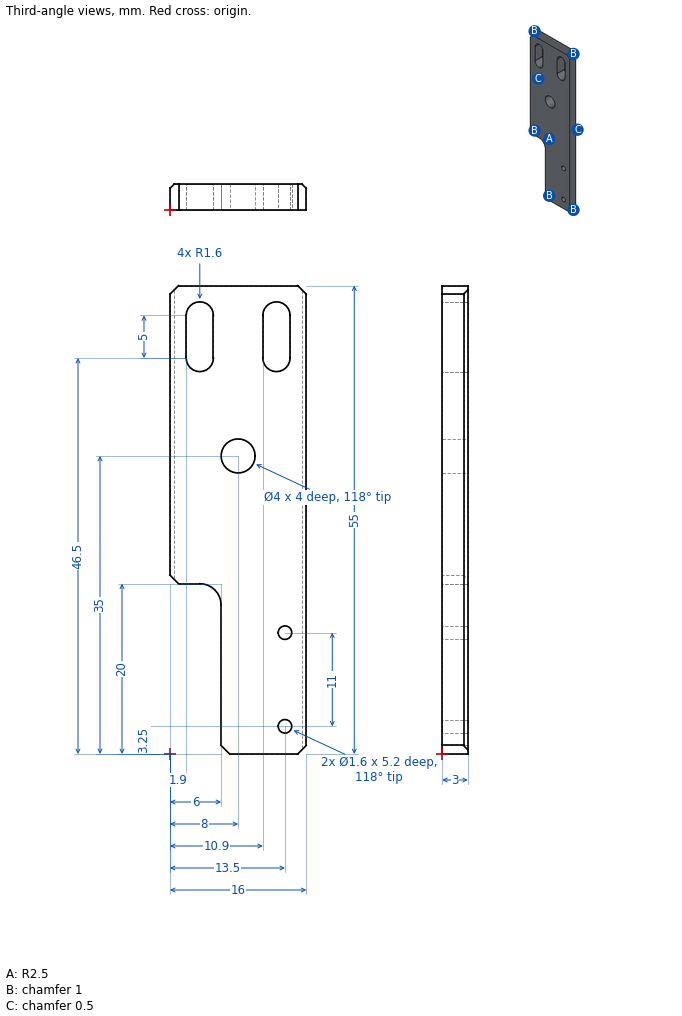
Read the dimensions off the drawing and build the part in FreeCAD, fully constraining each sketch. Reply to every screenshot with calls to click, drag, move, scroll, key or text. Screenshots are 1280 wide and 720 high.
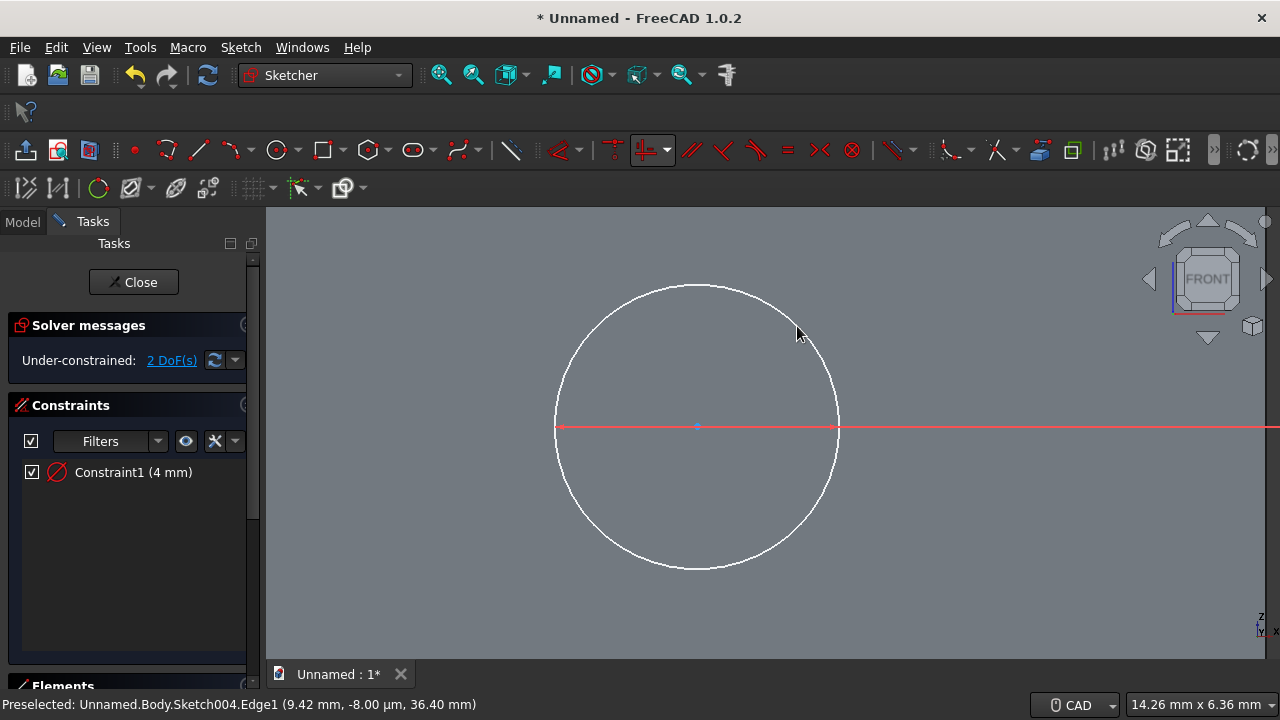
click(558, 150)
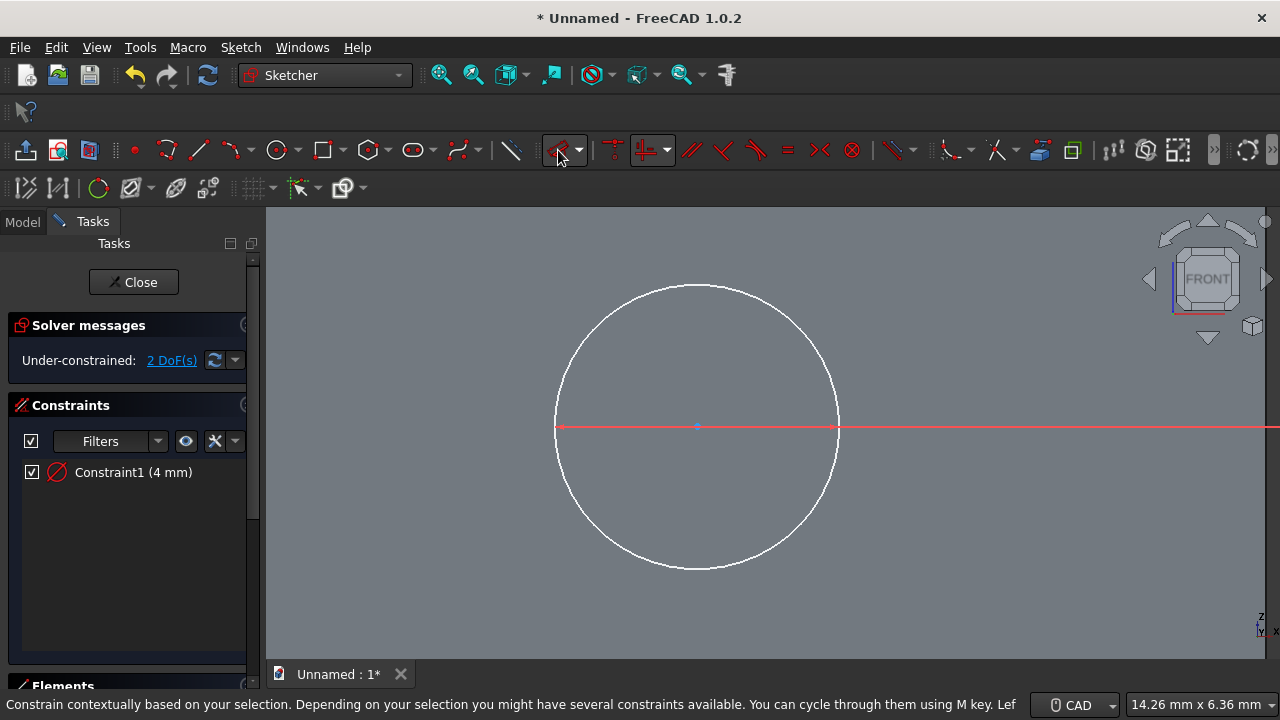
click(697, 427)
click(495, 393)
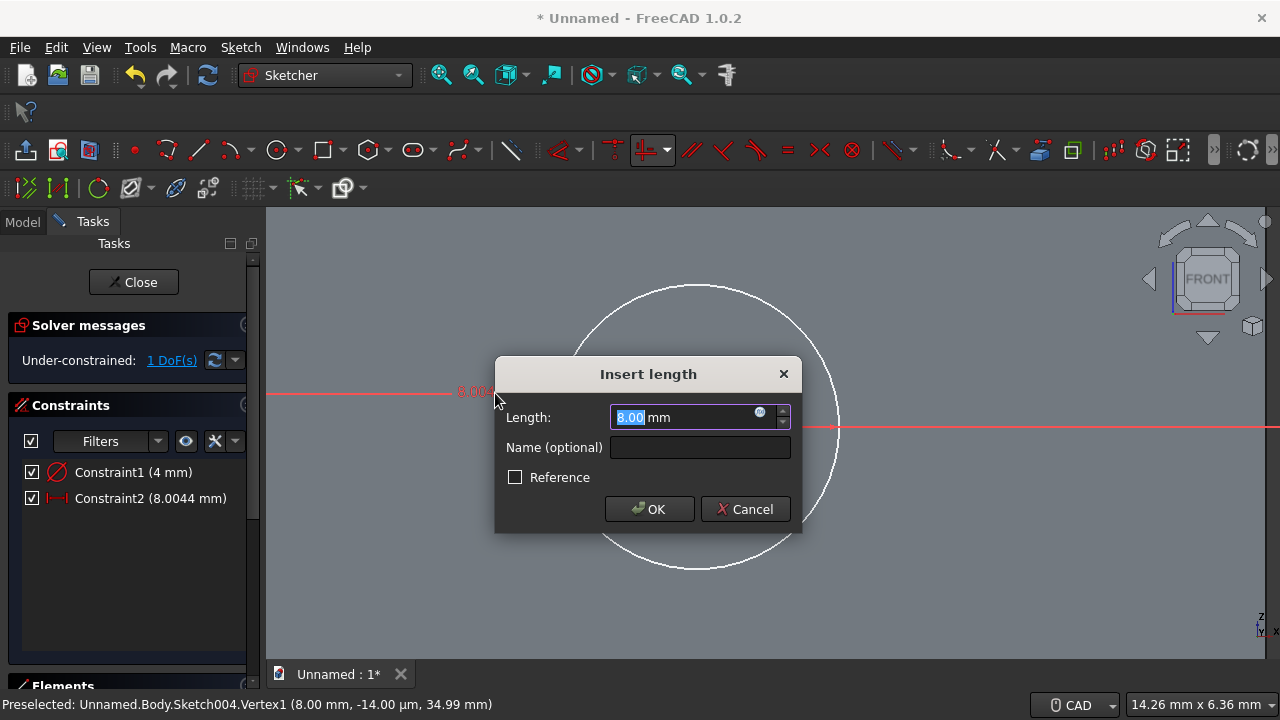
text(8)
key(Return)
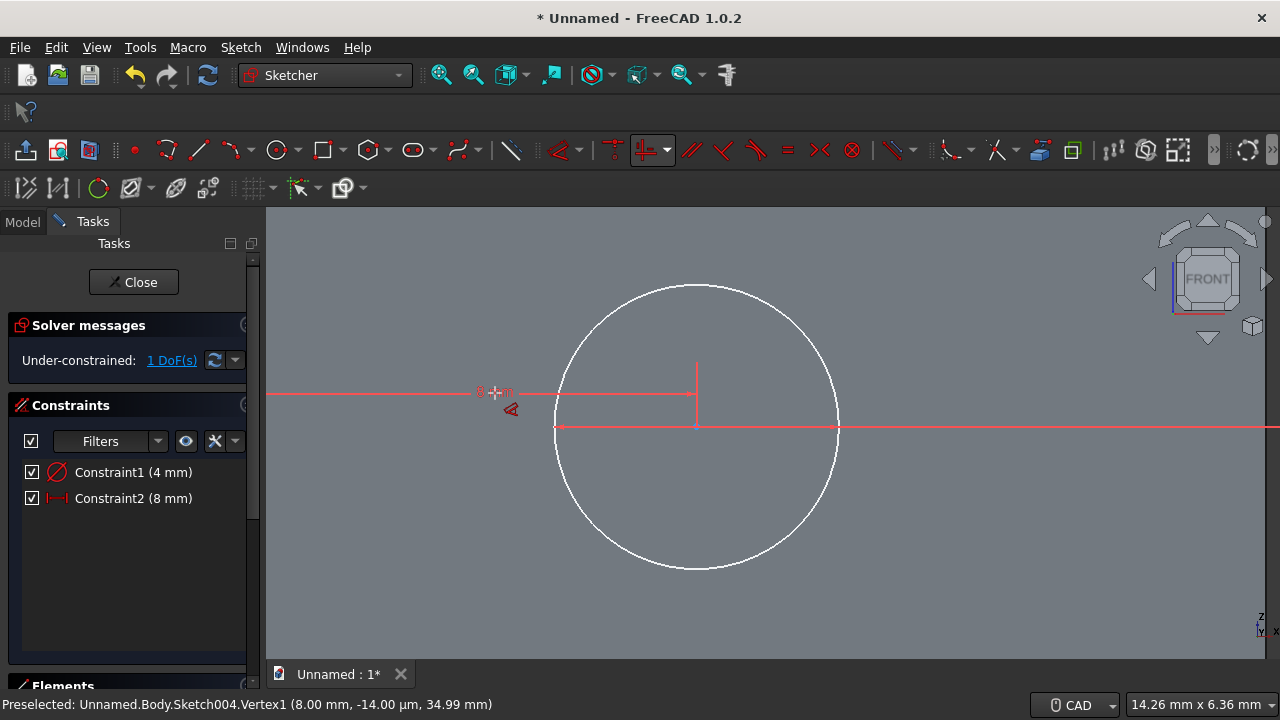
click(697, 427)
click(731, 529)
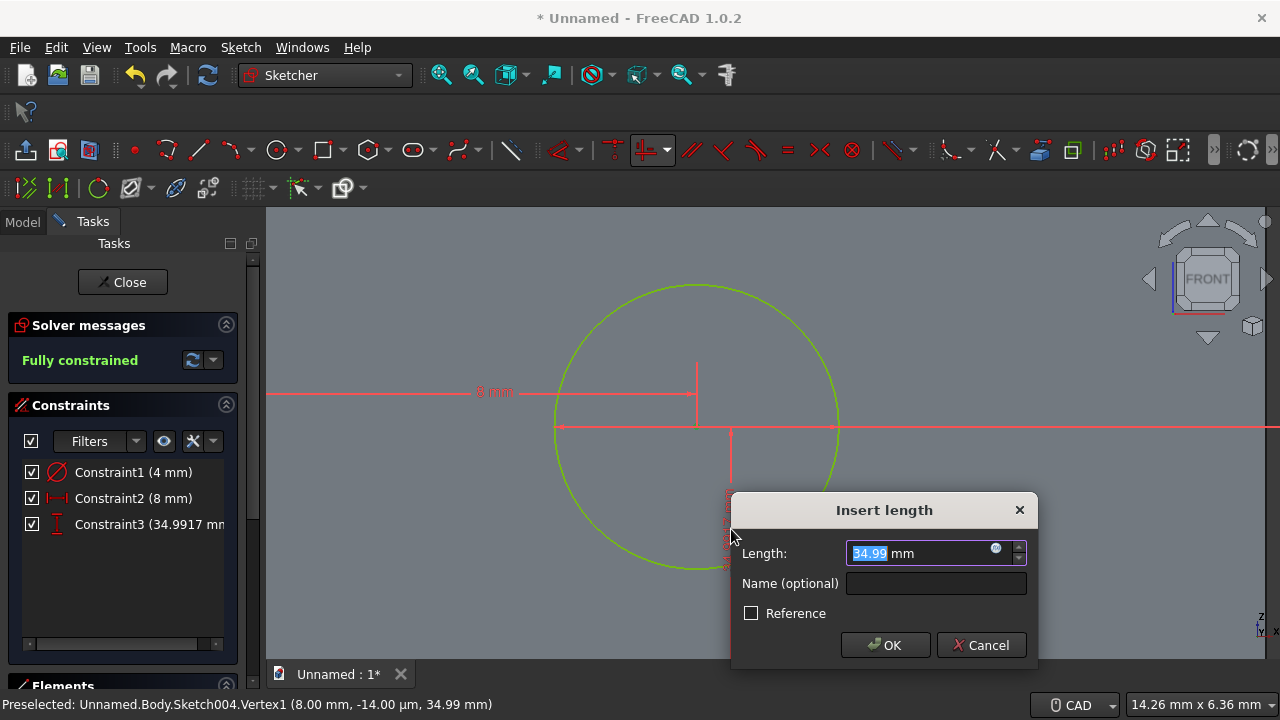
text(35)
key(Return)
key(Escape)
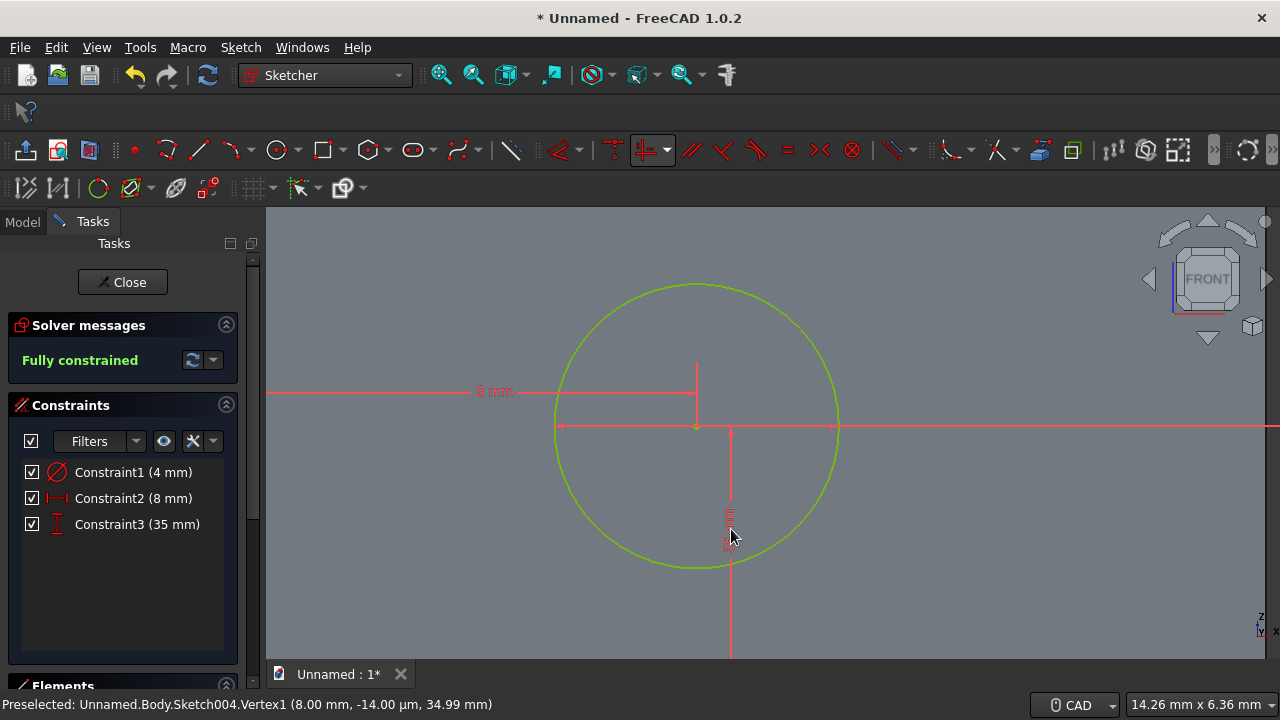
click(123, 282)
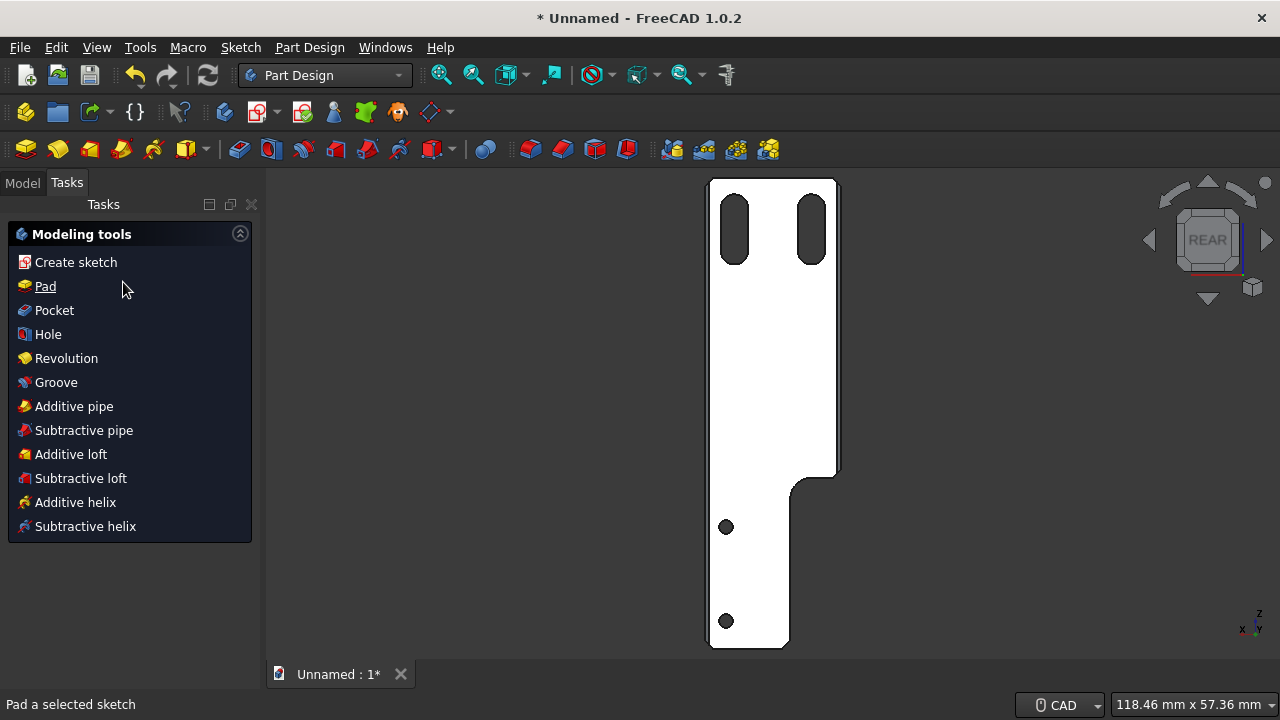
click(272, 150)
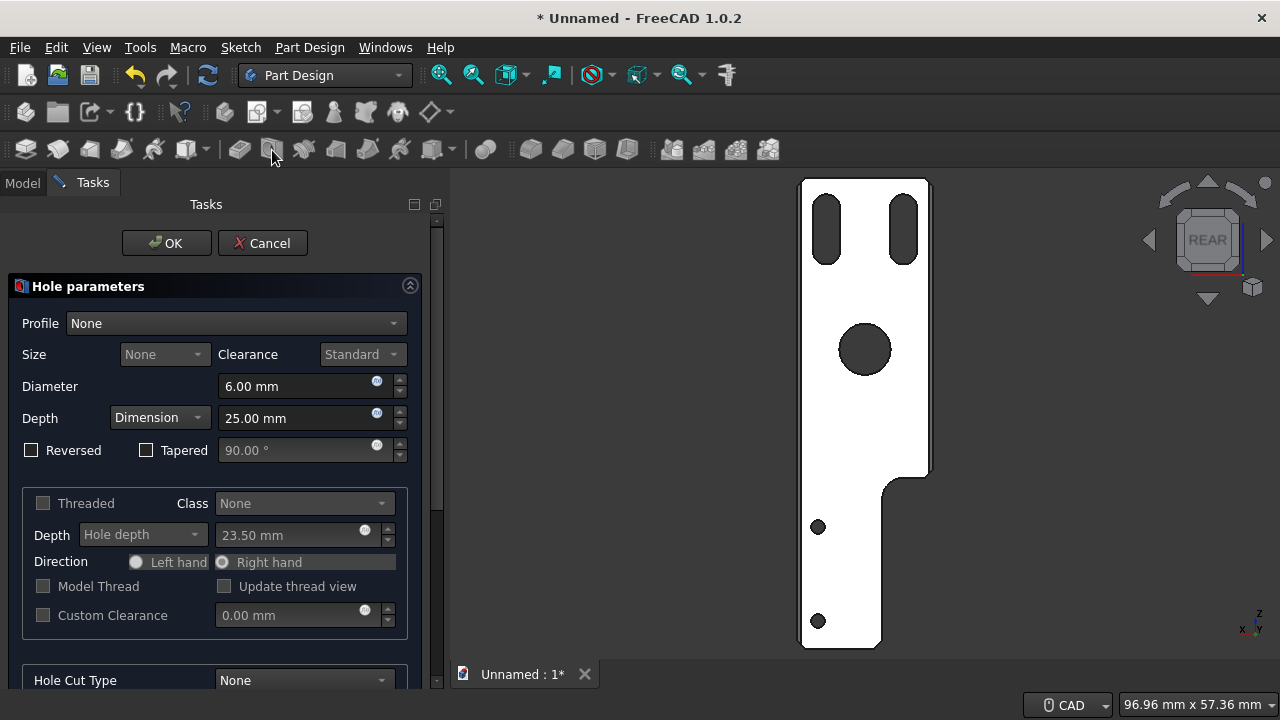
triple_click(305, 386)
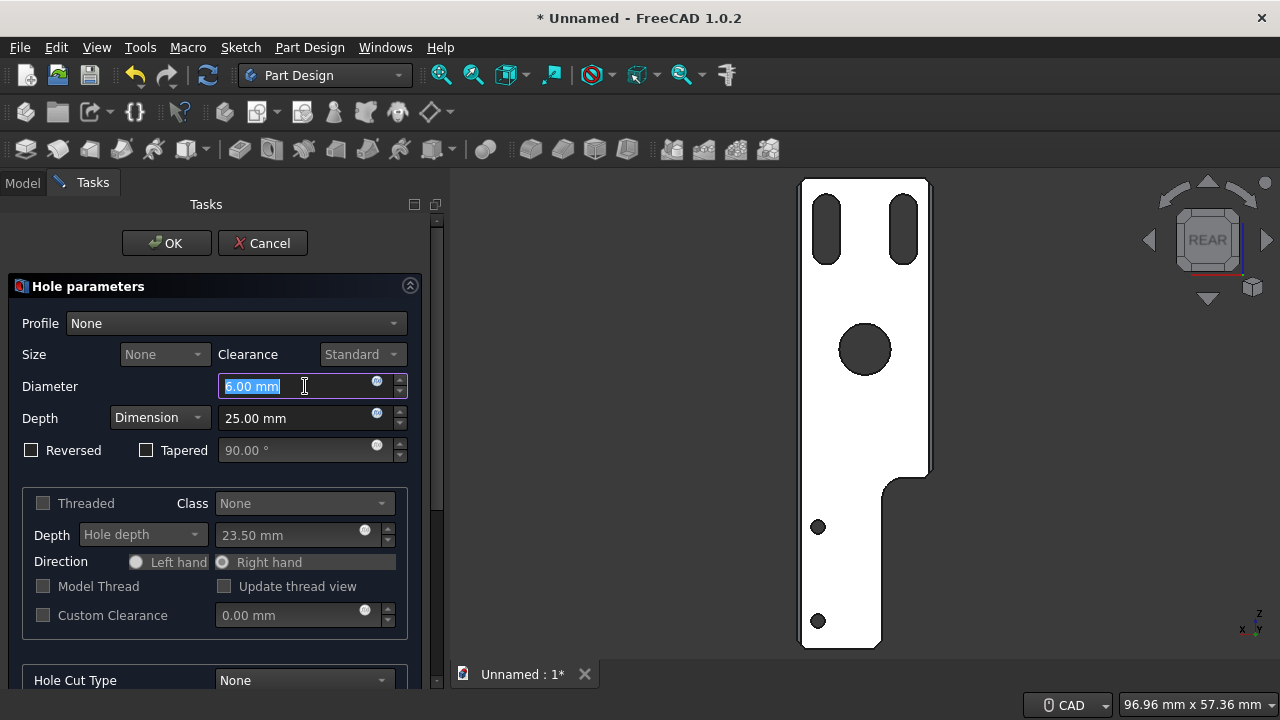
text(4)
key(Tab)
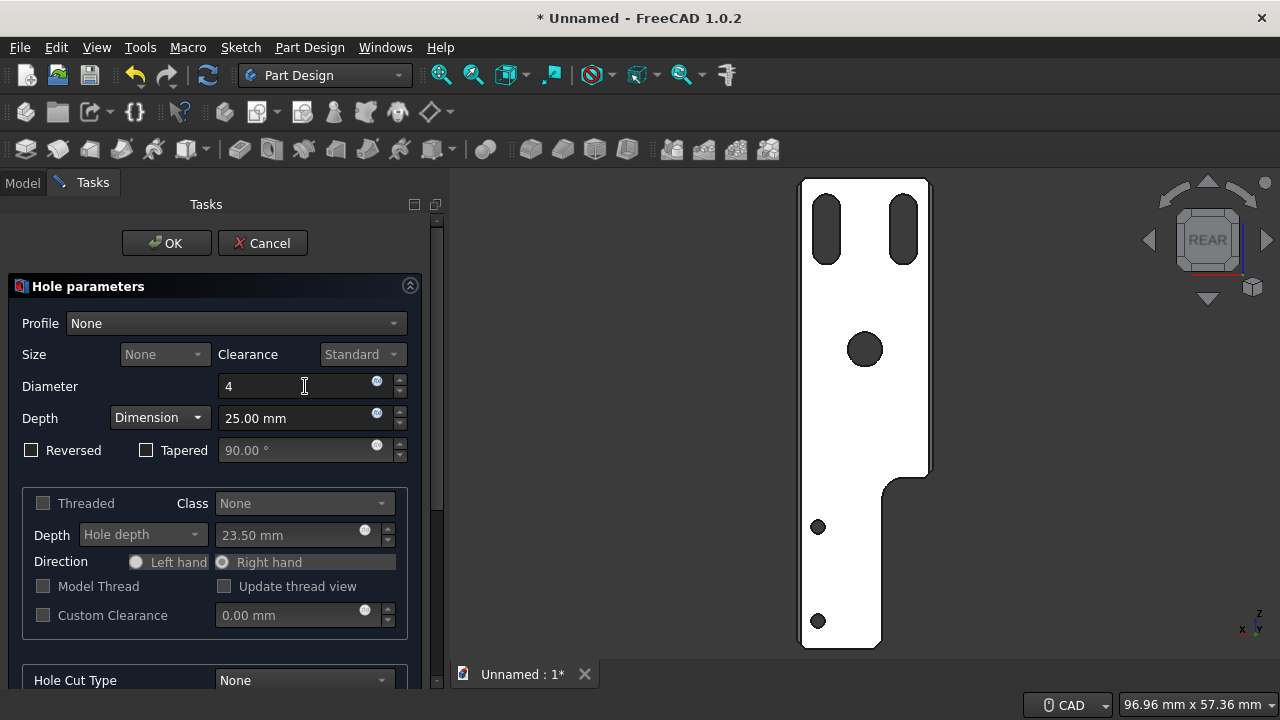
triple_click(305, 418)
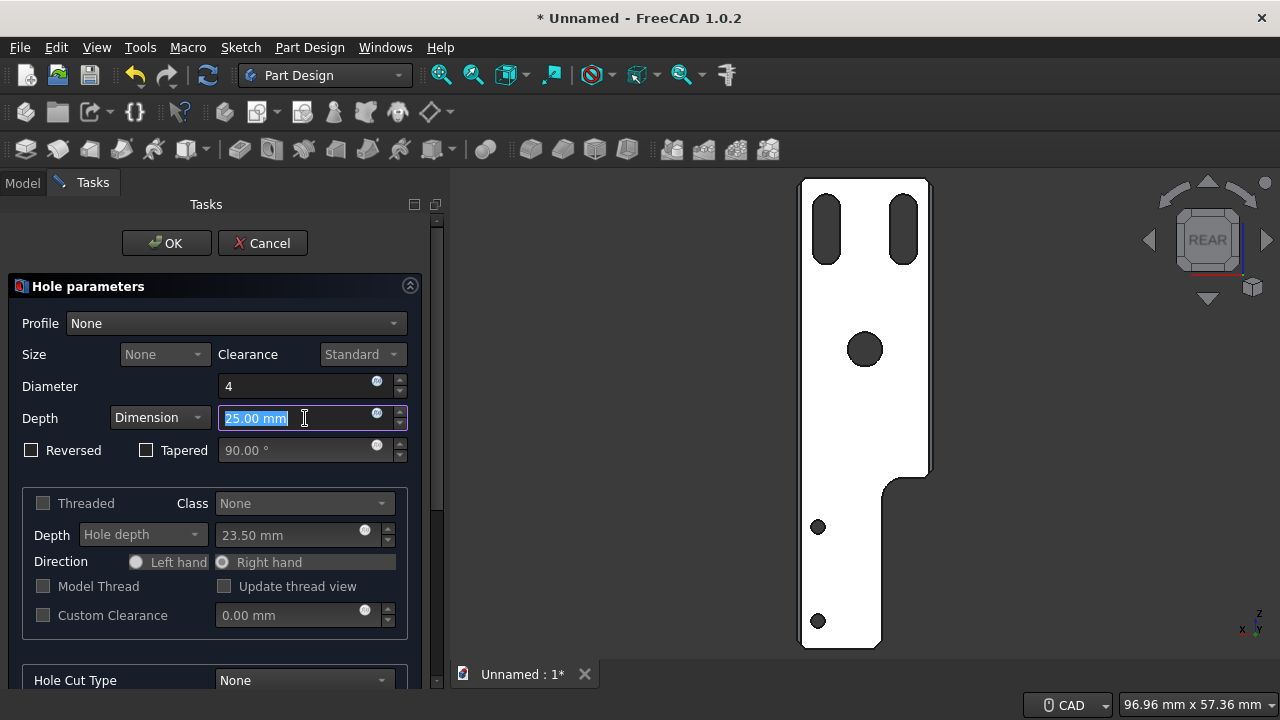
text(4)
key(Tab)